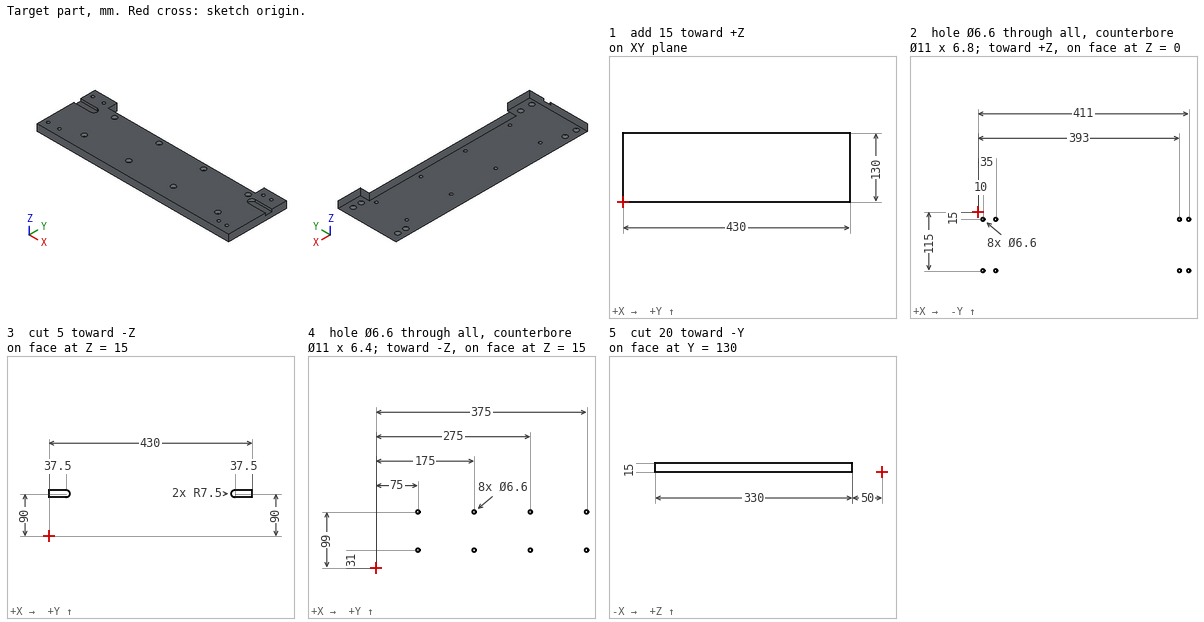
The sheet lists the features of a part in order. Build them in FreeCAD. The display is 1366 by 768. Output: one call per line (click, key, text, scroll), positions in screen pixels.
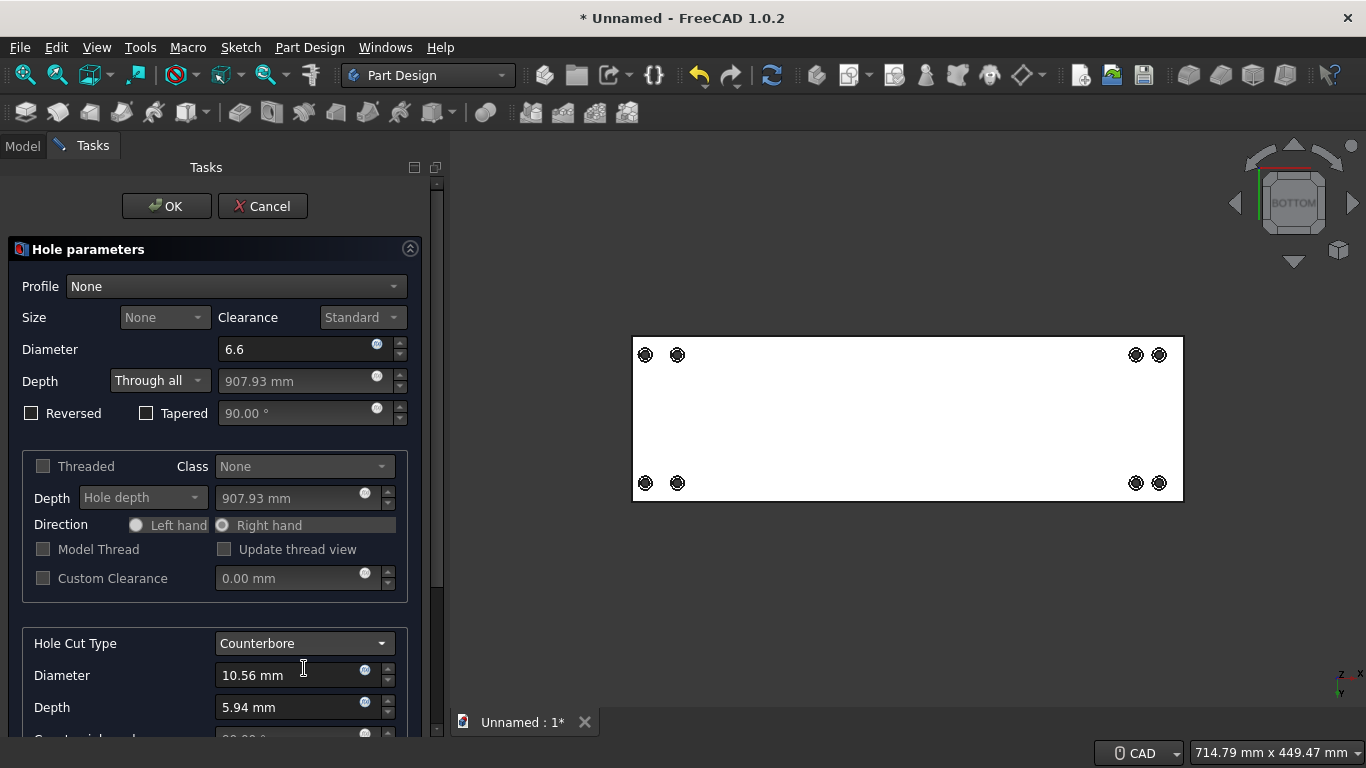
triple_click(298, 675)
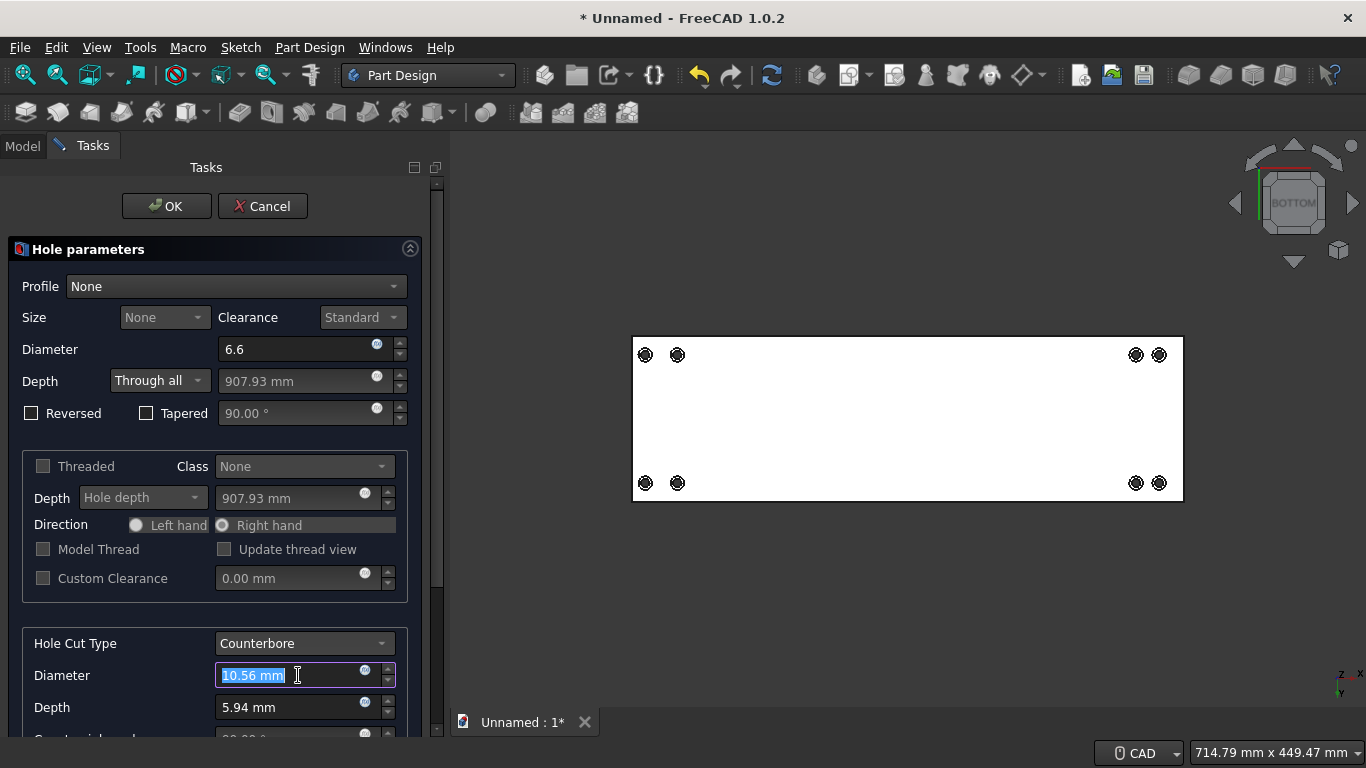
text(11)
key(Tab)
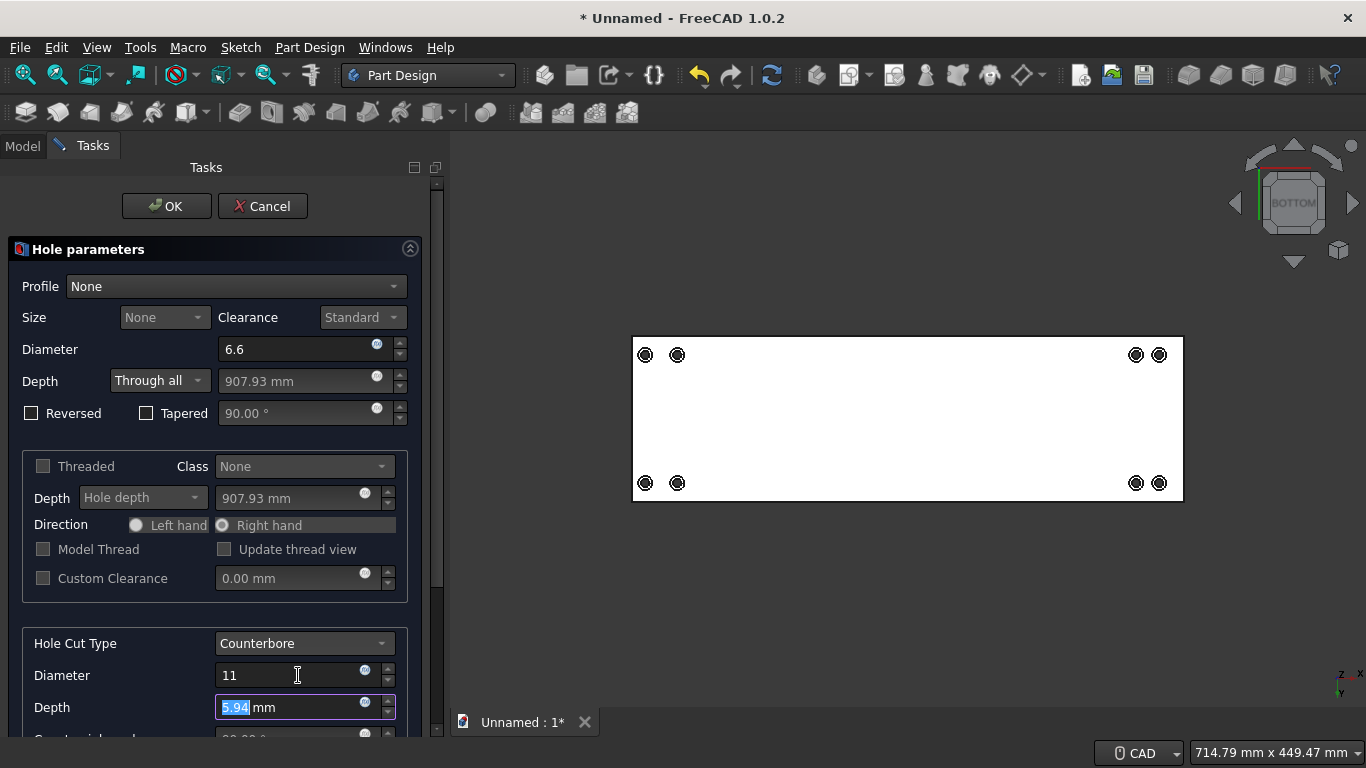
text(6.8)
key(Tab)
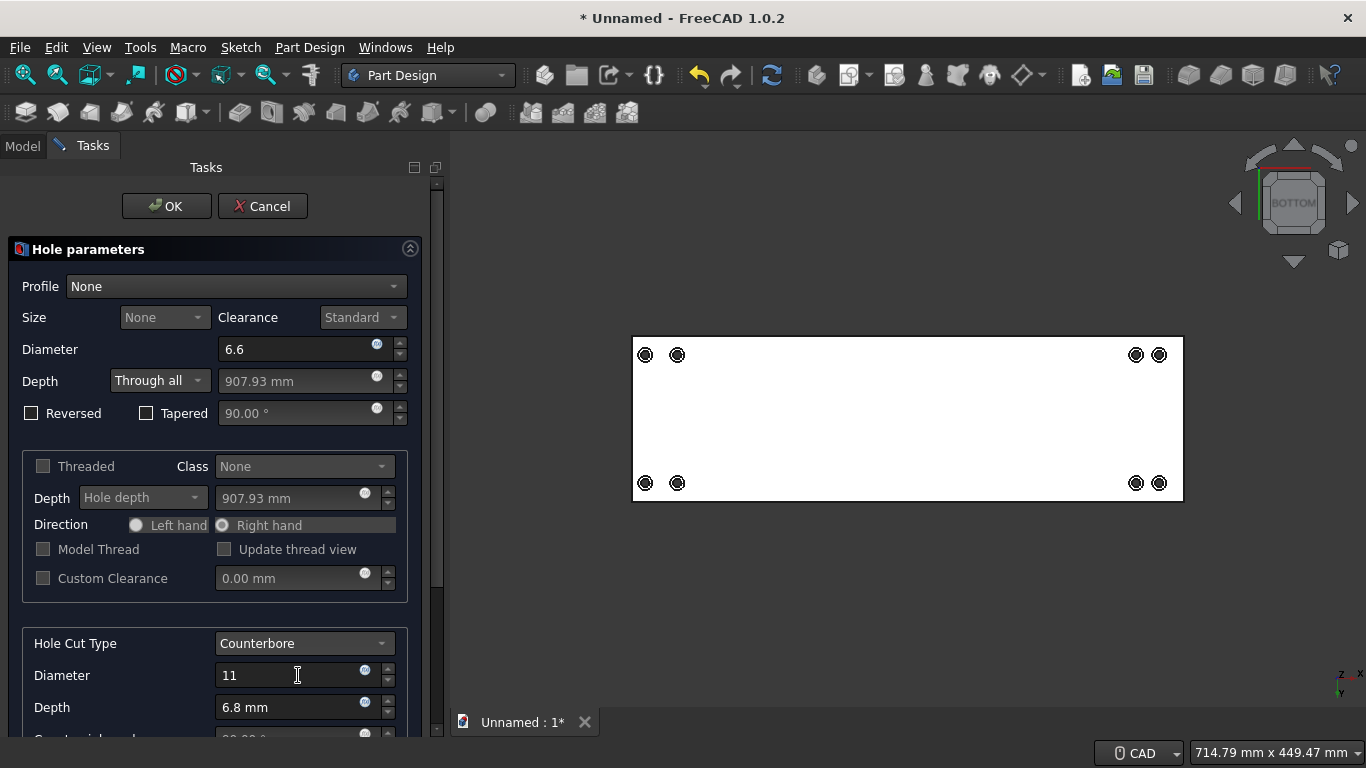
click(167, 206)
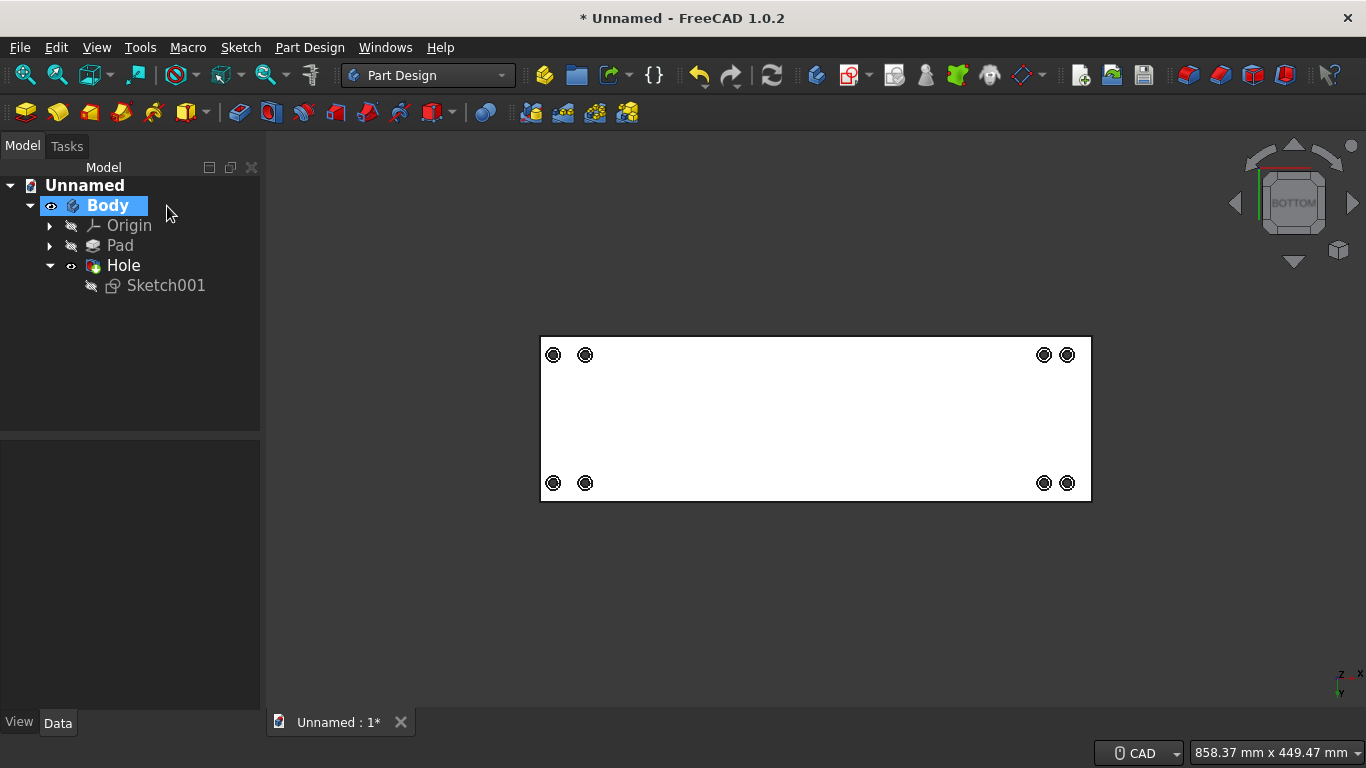
key(0)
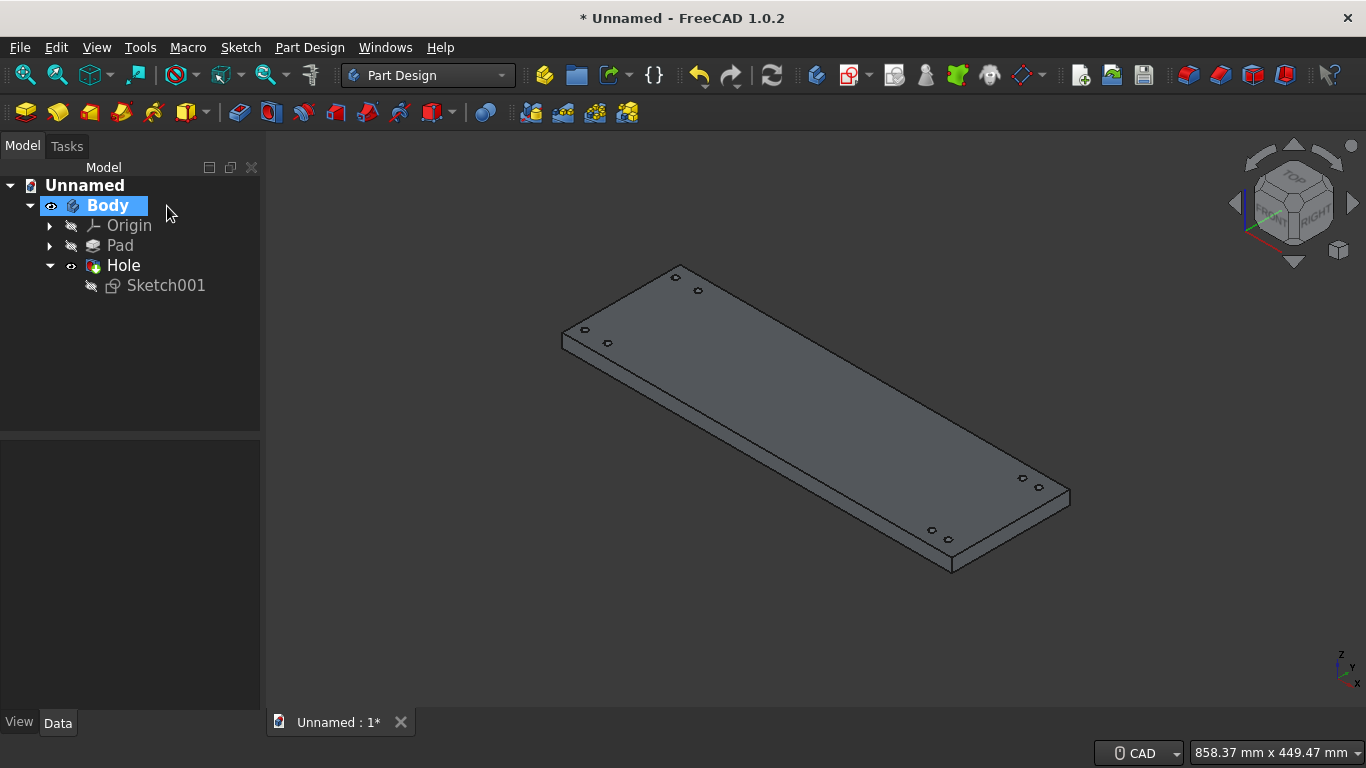
click(927, 474)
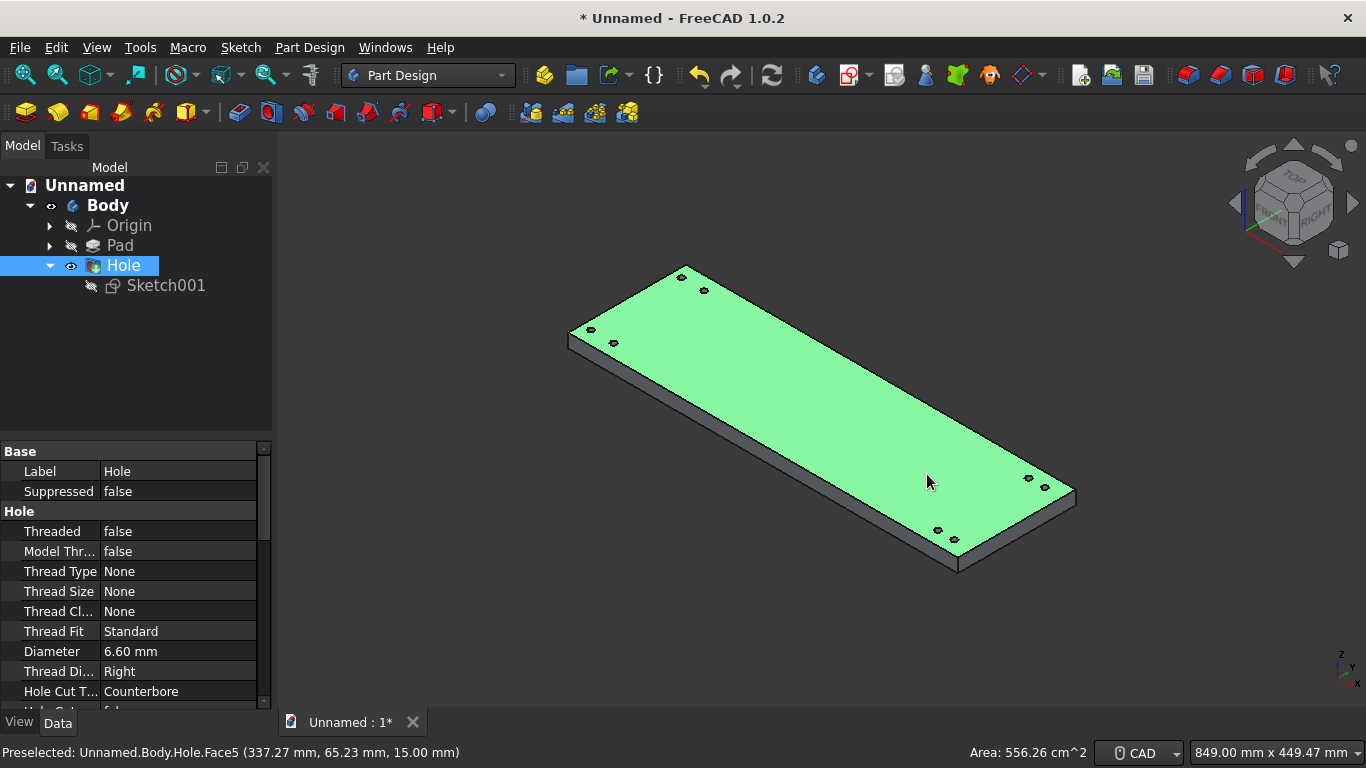
click(850, 76)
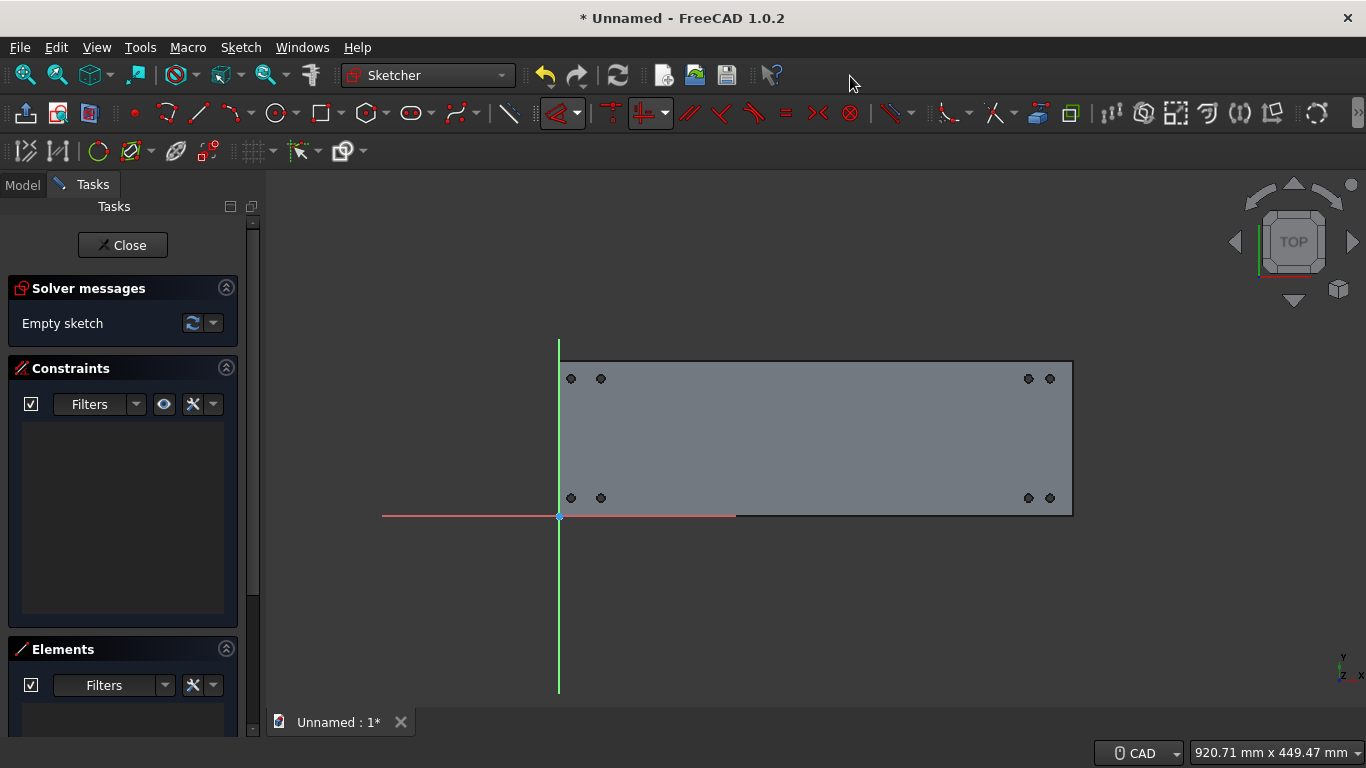
key(g)
key(m)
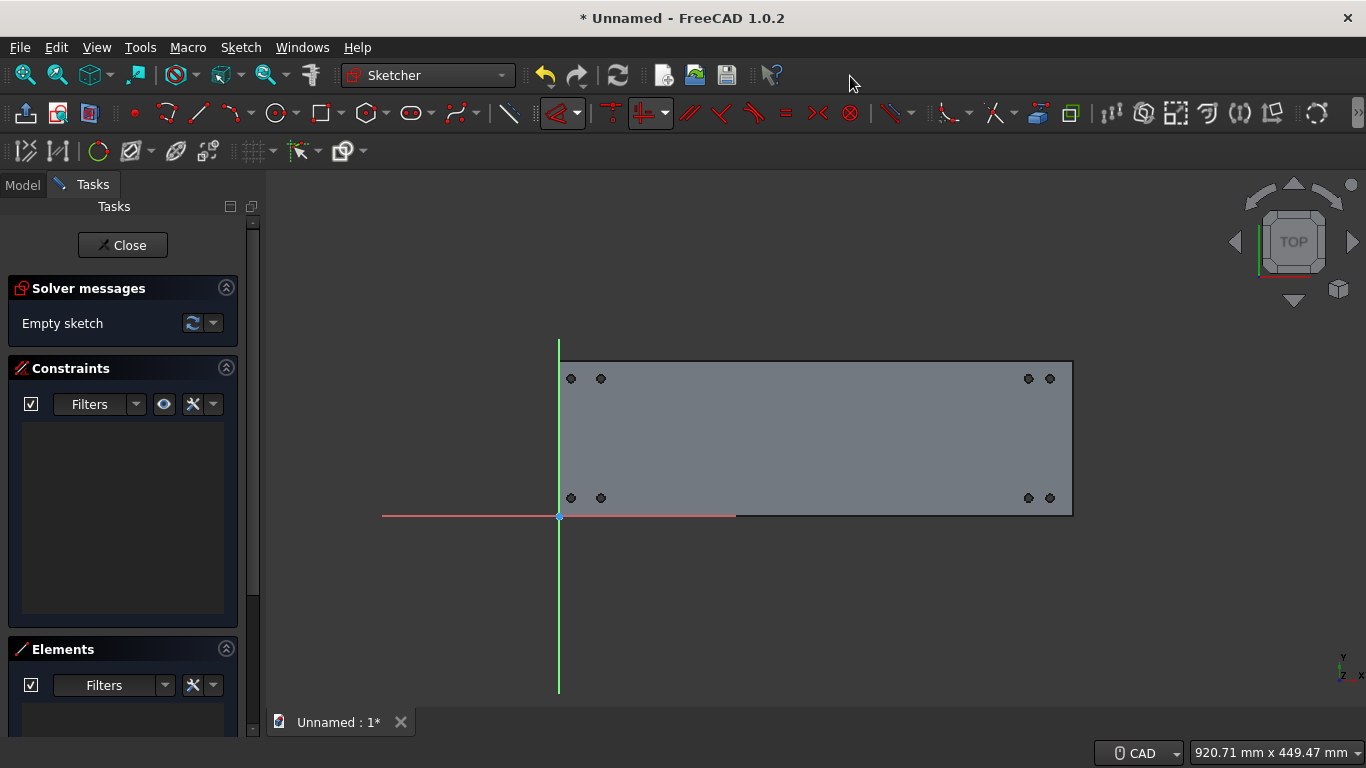
click(1028, 418)
click(1073, 418)
click(1073, 400)
click(1028, 400)
right_click(1028, 400)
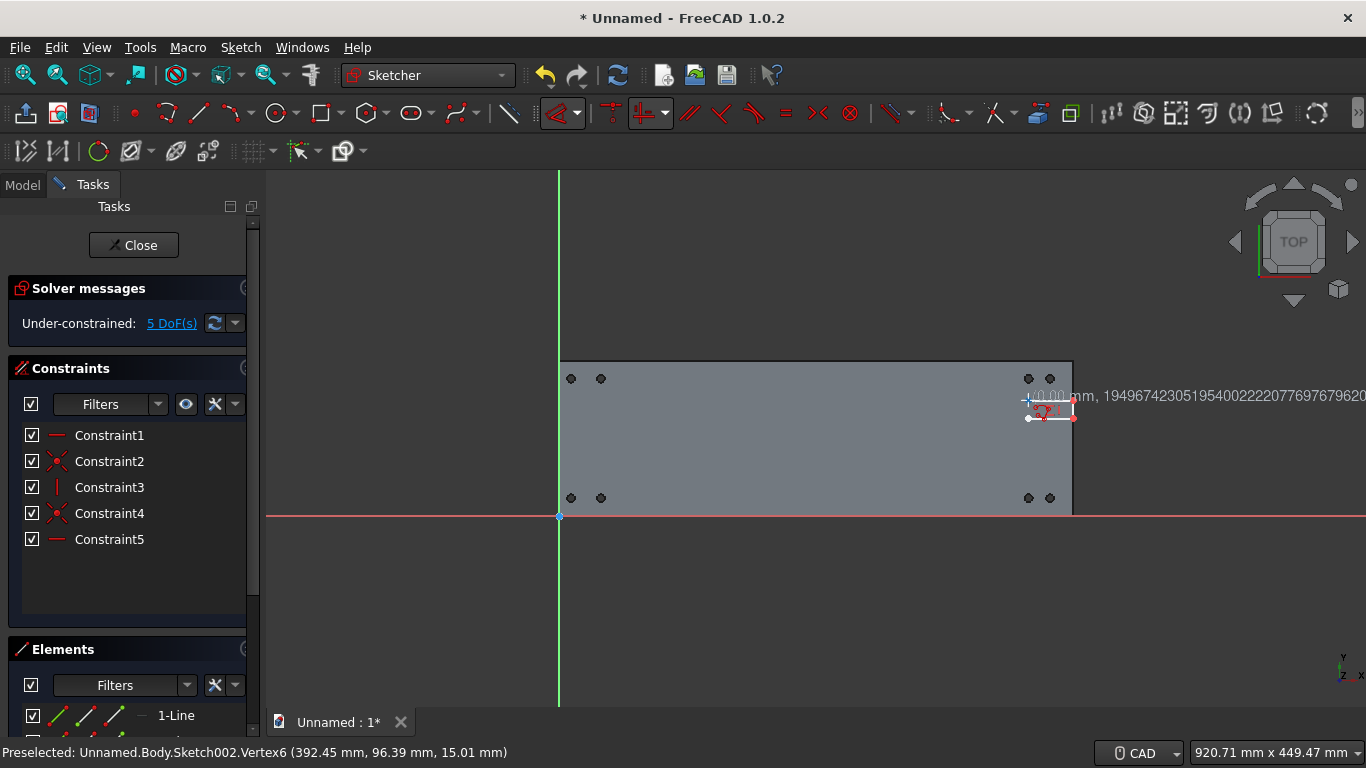
click(232, 114)